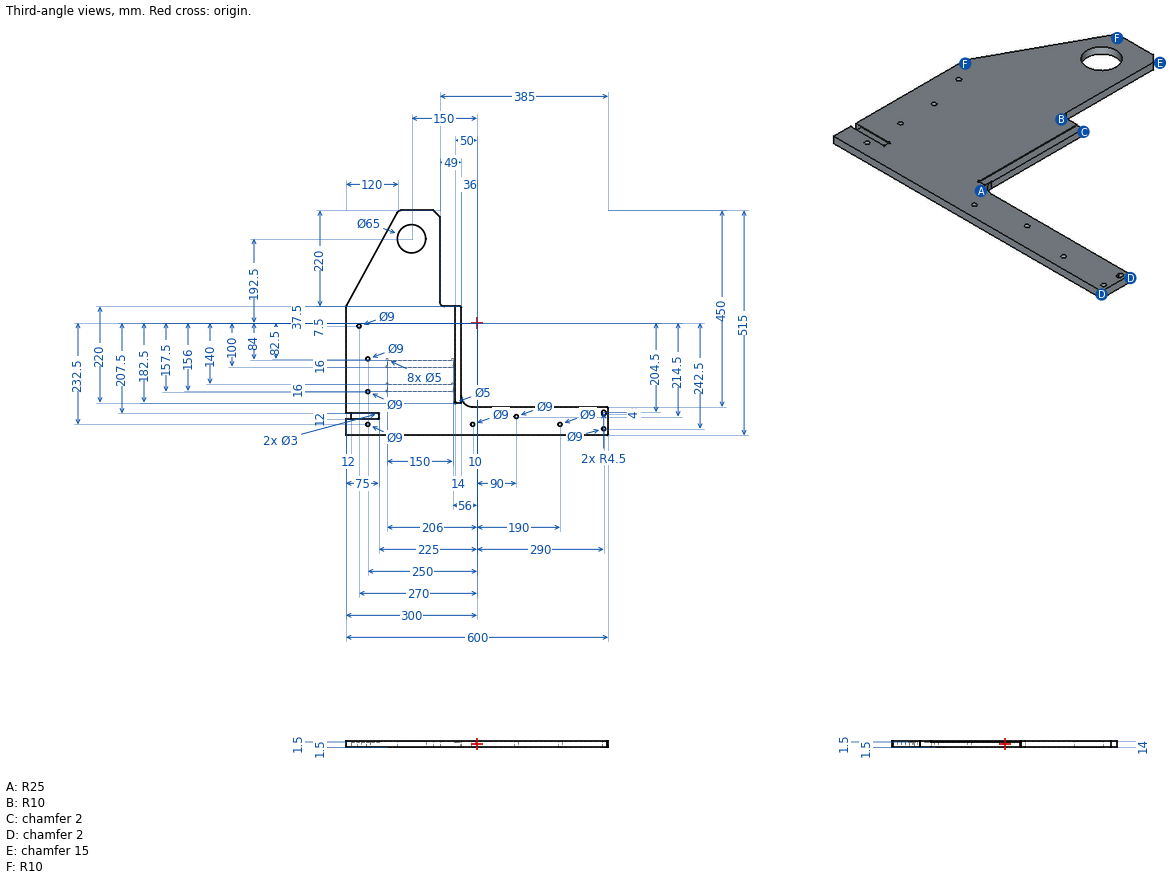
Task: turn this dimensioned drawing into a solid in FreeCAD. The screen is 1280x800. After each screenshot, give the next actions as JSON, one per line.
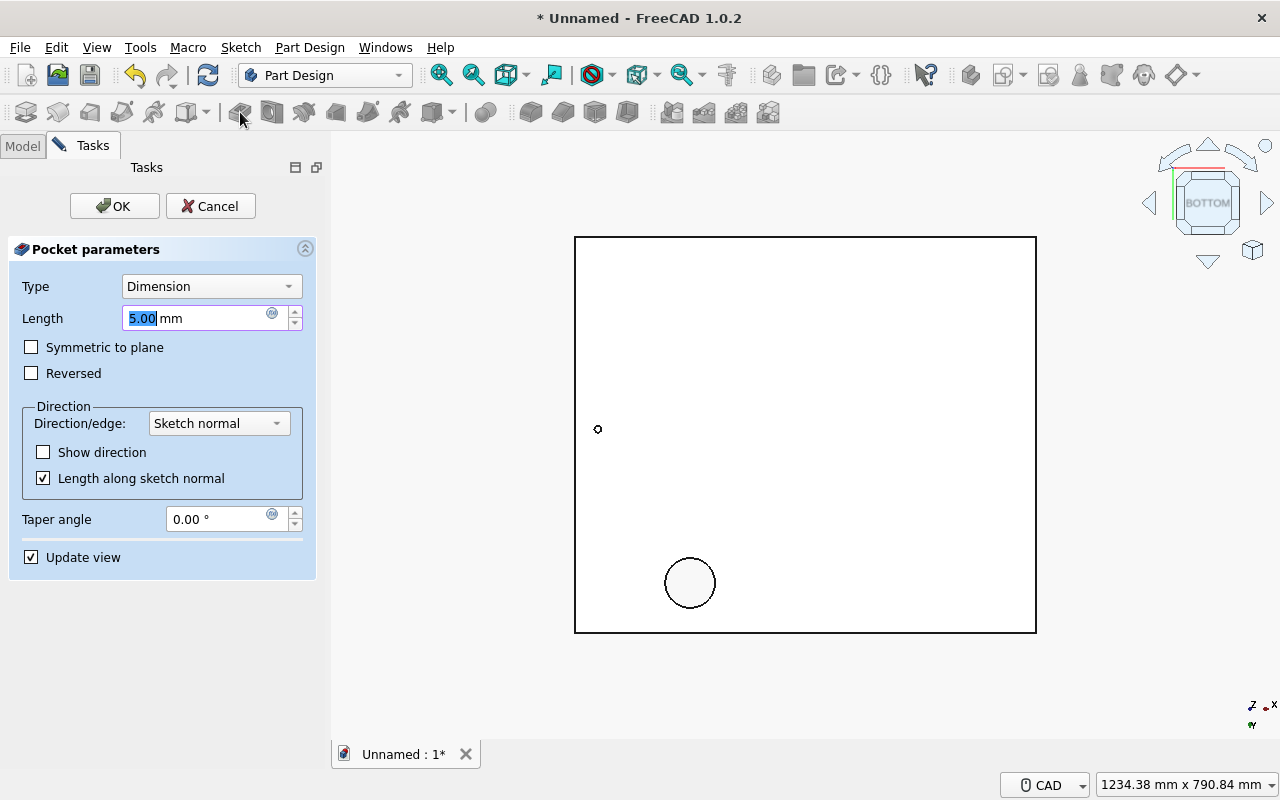
{"action": "left_click", "coordinate": [212, 286]}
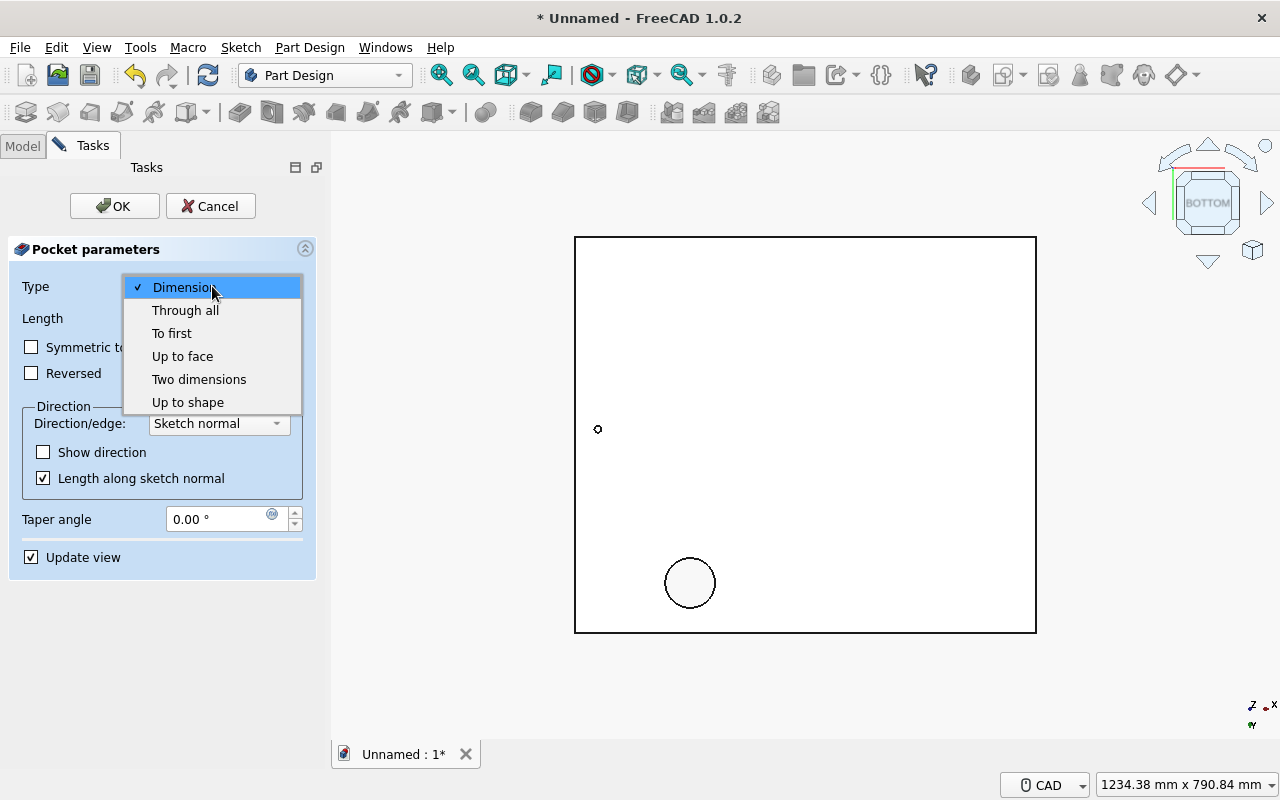
{"action": "left_click", "coordinate": [212, 334]}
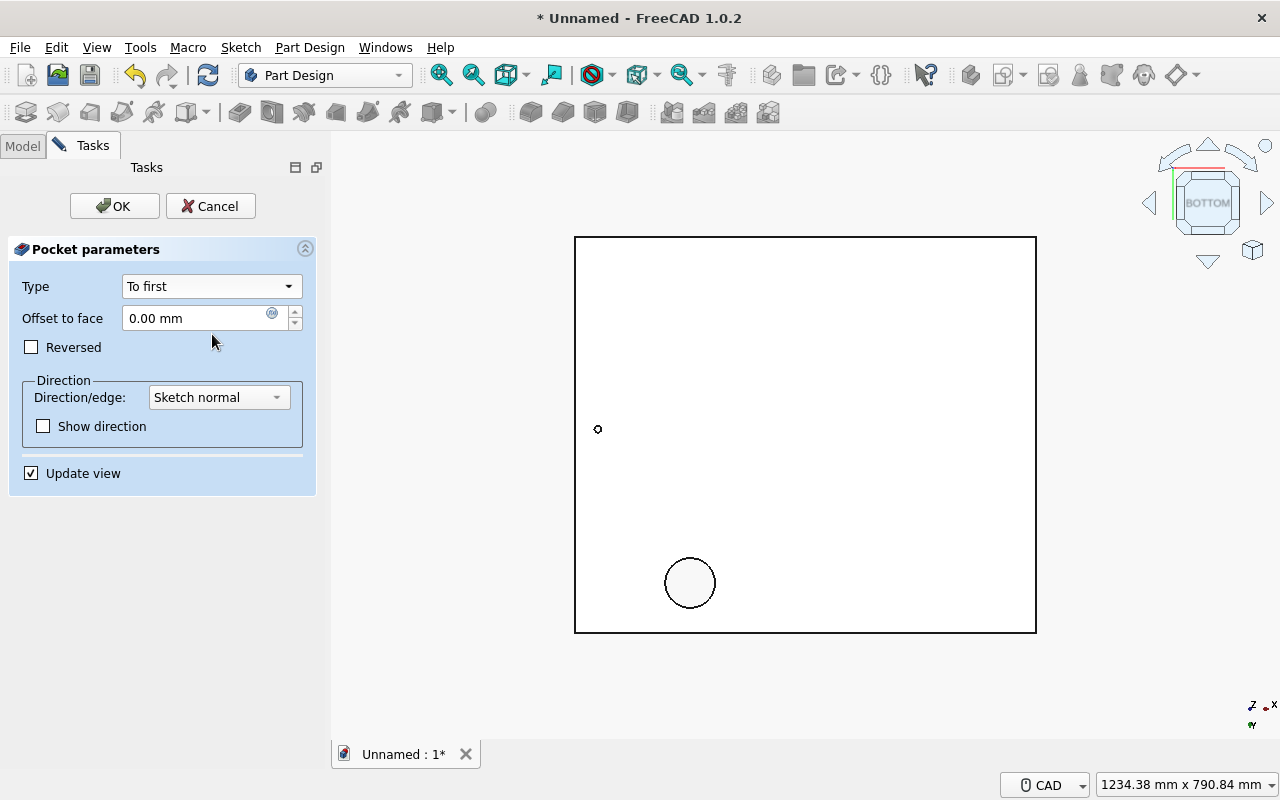
{"action": "left_click", "coordinate": [115, 206]}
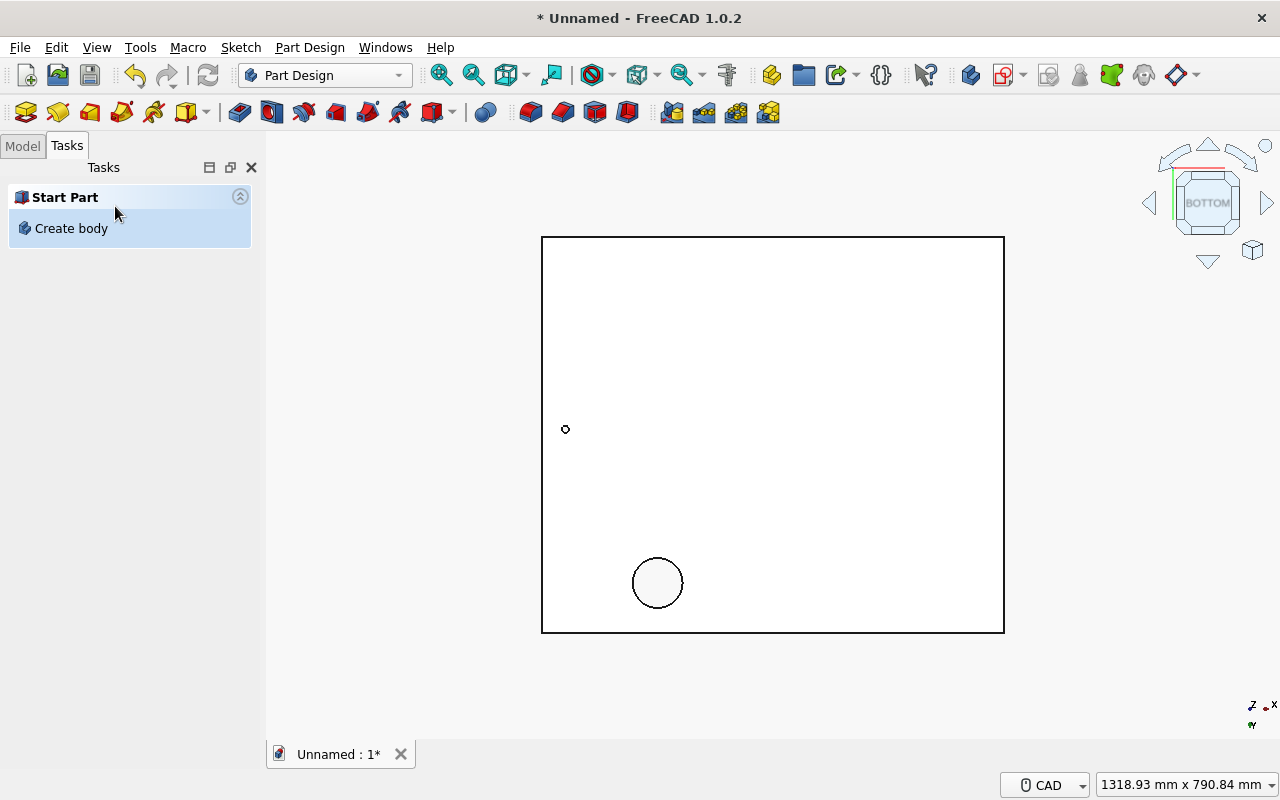
{"action": "left_click", "coordinate": [839, 434]}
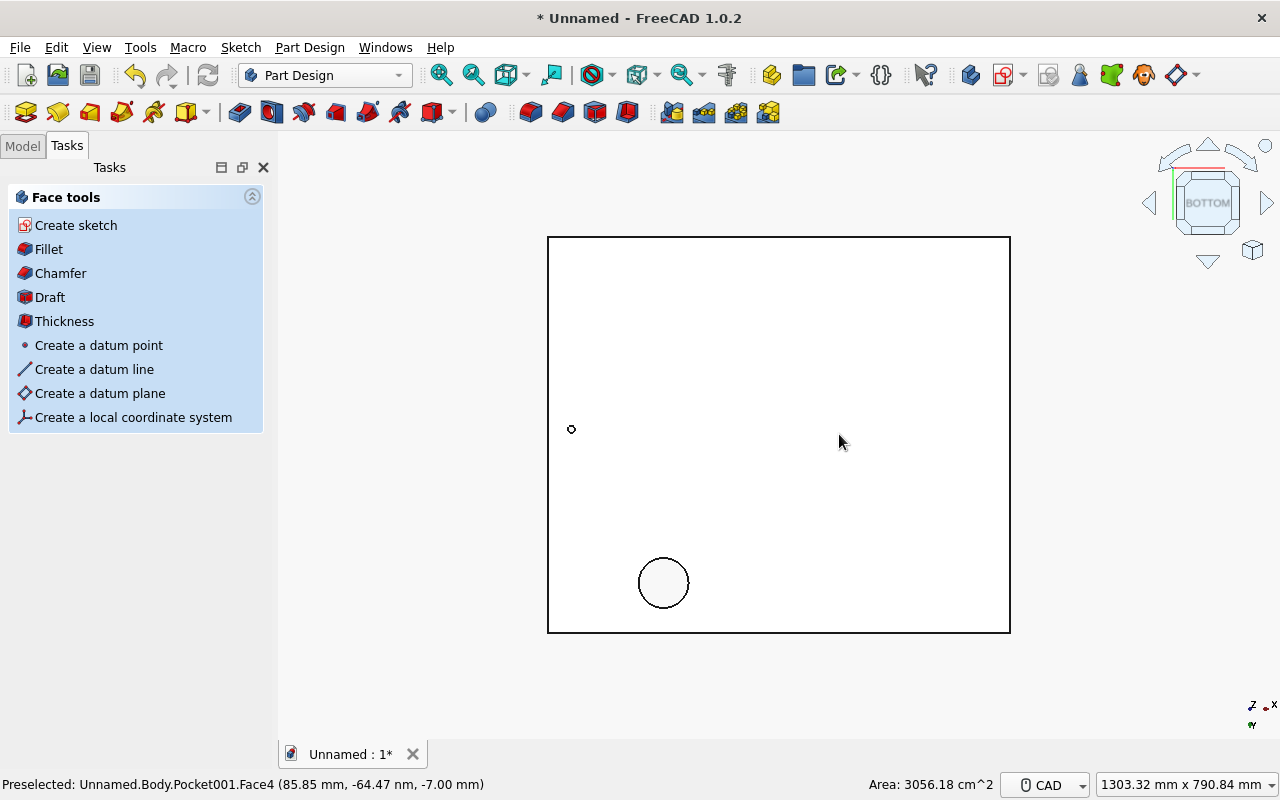
{"action": "left_click", "coordinate": [1004, 76]}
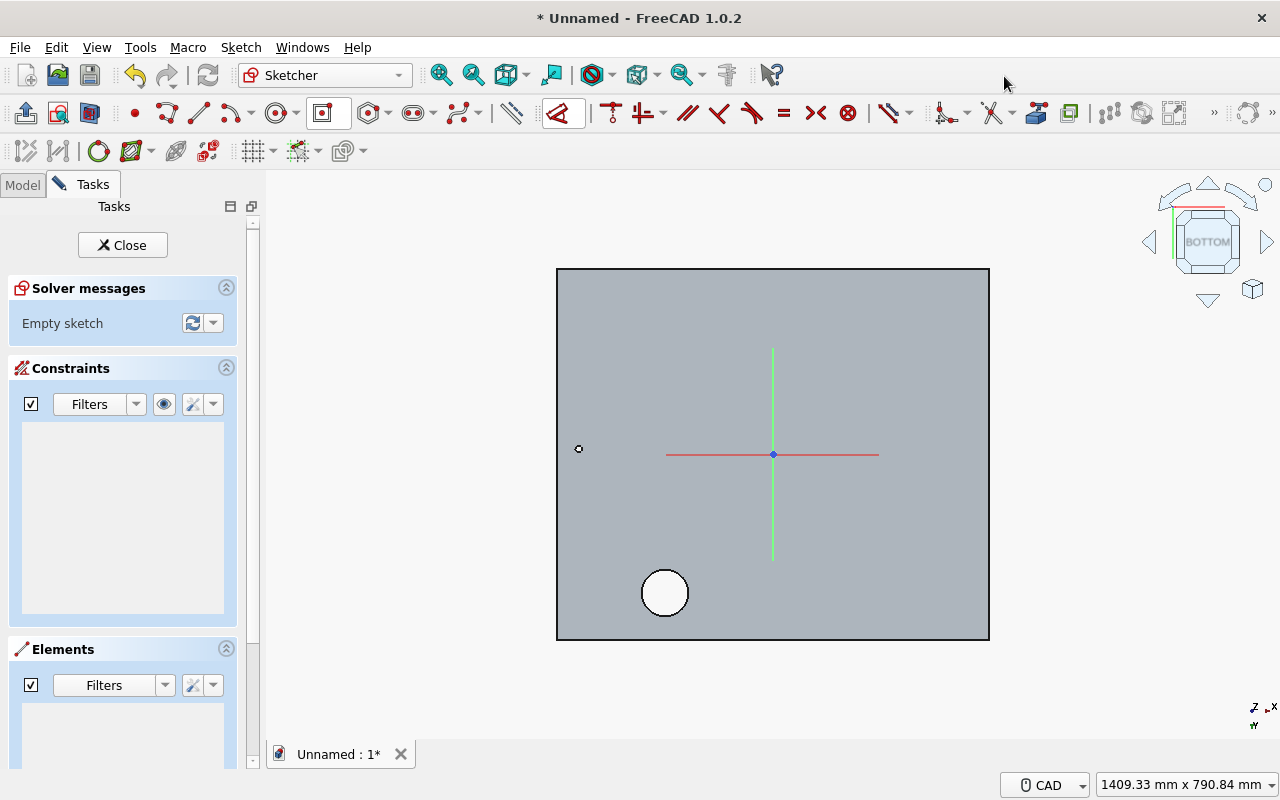
{"action": "scroll", "coordinate": [587, 392], "scroll_direction": "up", "scroll_amount": 15}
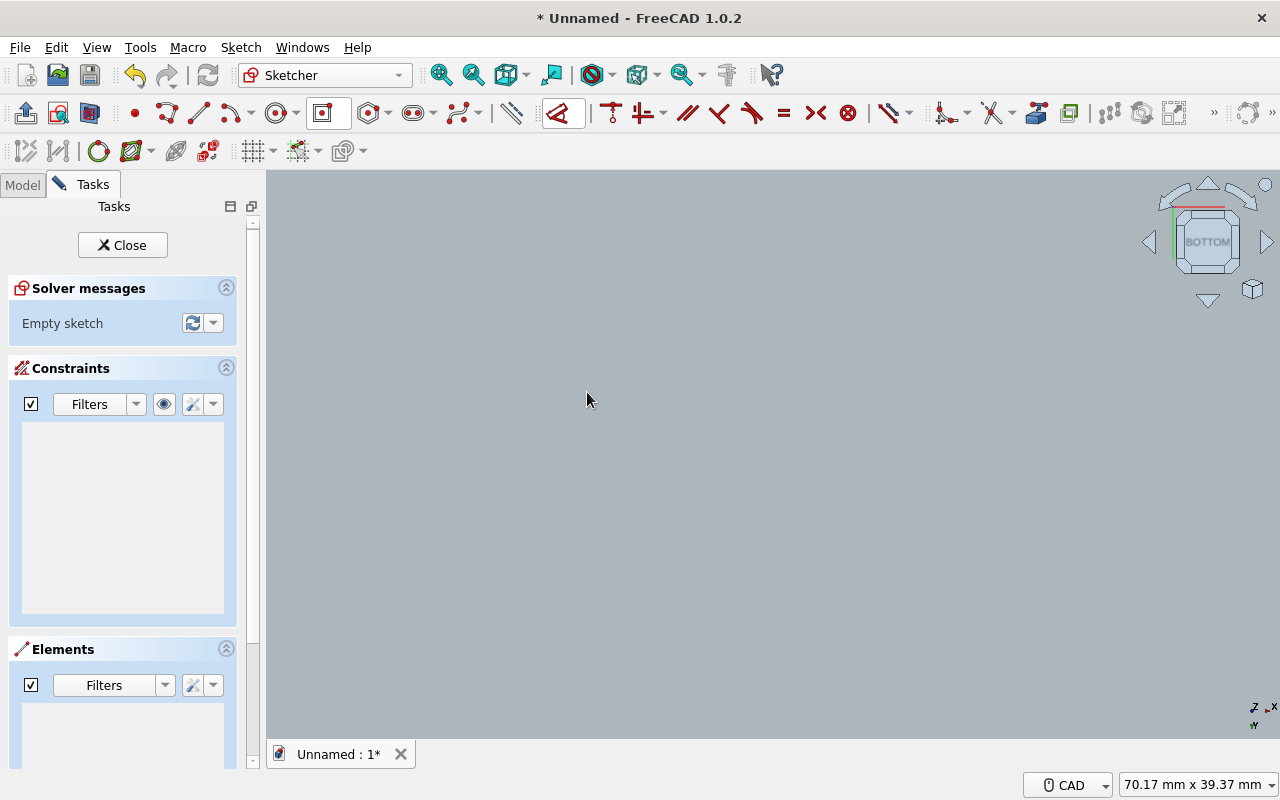
{"action": "scroll", "coordinate": [704, 444], "scroll_direction": "up", "scroll_amount": 5}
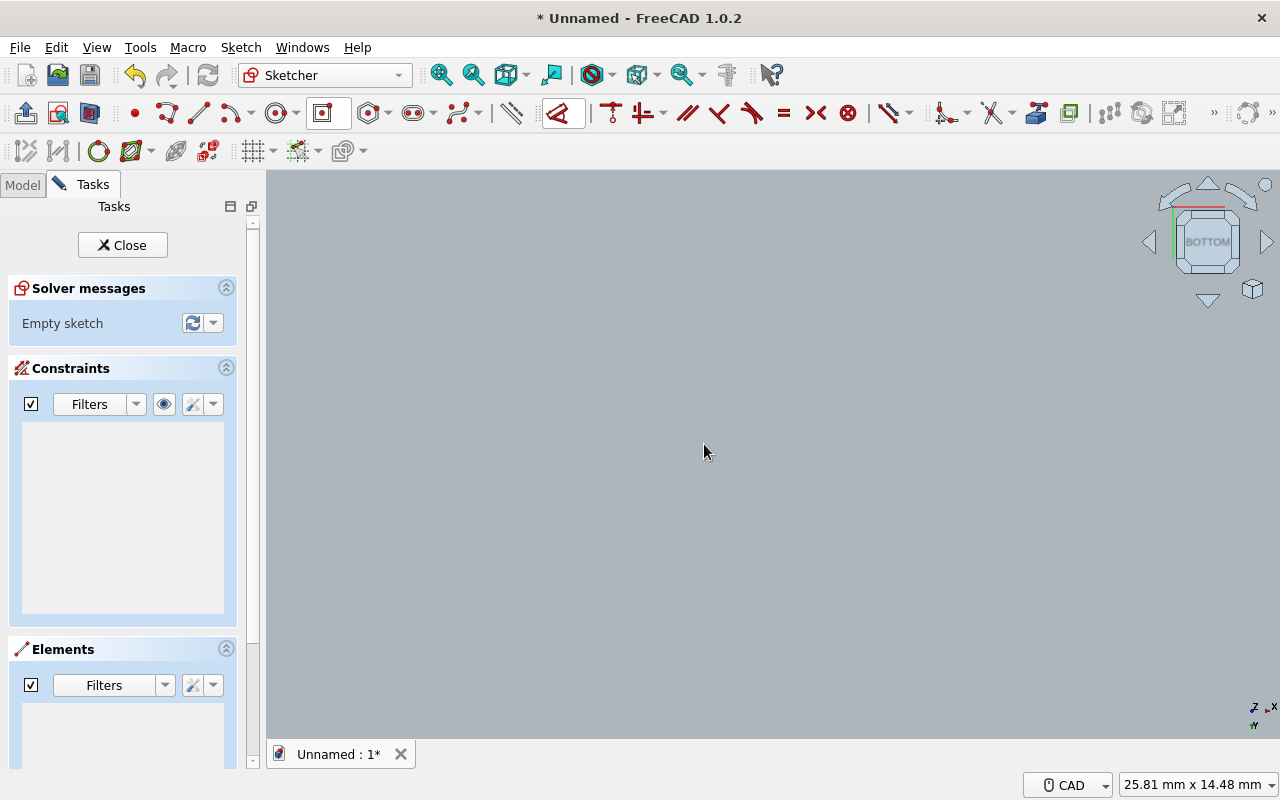
{"action": "left_click", "coordinate": [276, 114]}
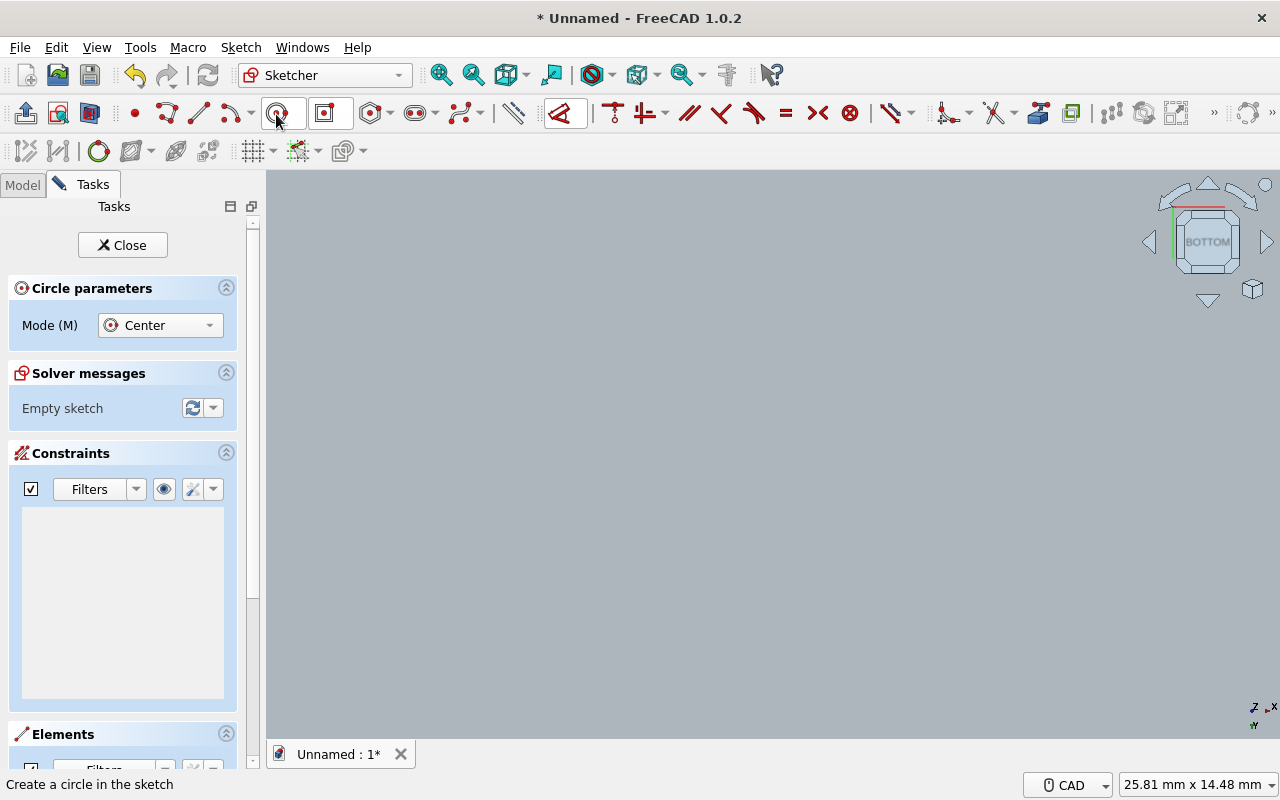
{"action": "left_click", "coordinate": [703, 453]}
{"action": "mouse_move", "coordinate": [828, 328]}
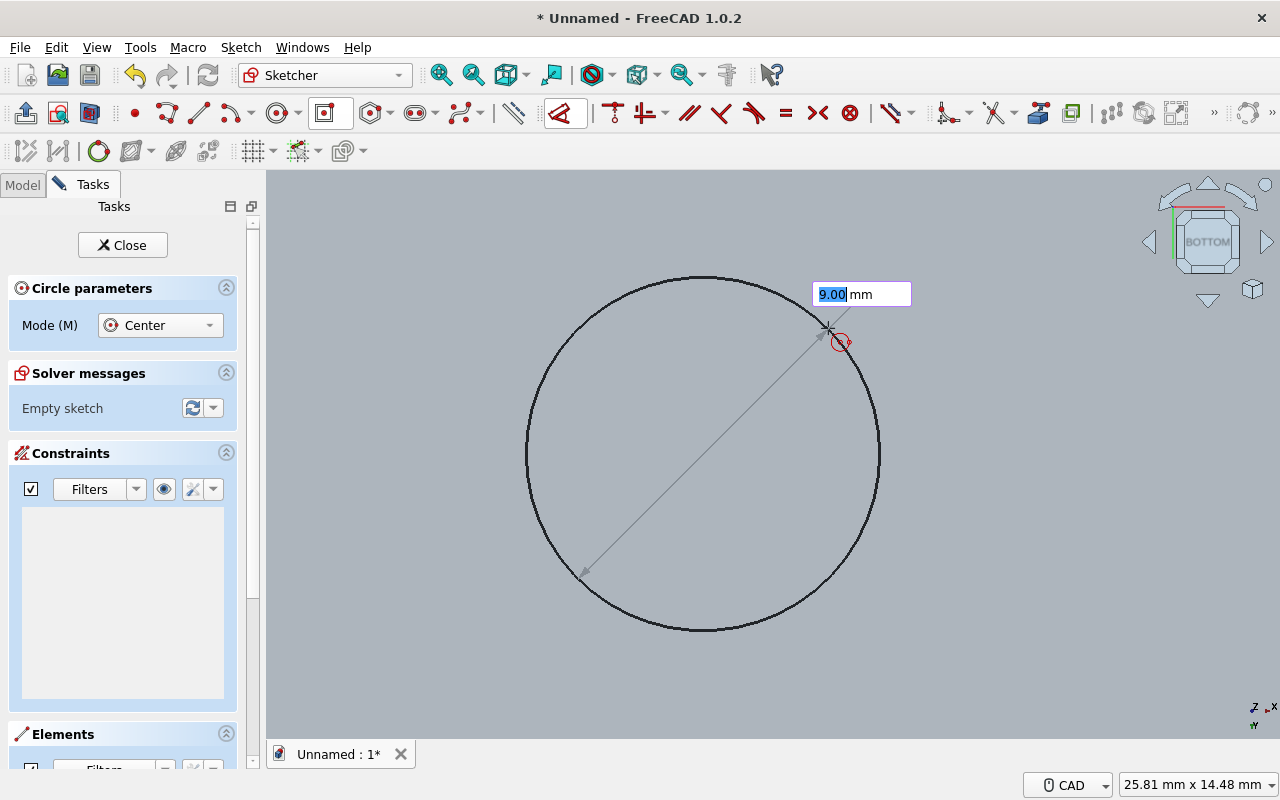
{"action": "type", "text": "9"}
{"action": "key", "text": "Return"}
{"action": "key", "text": "Escape"}